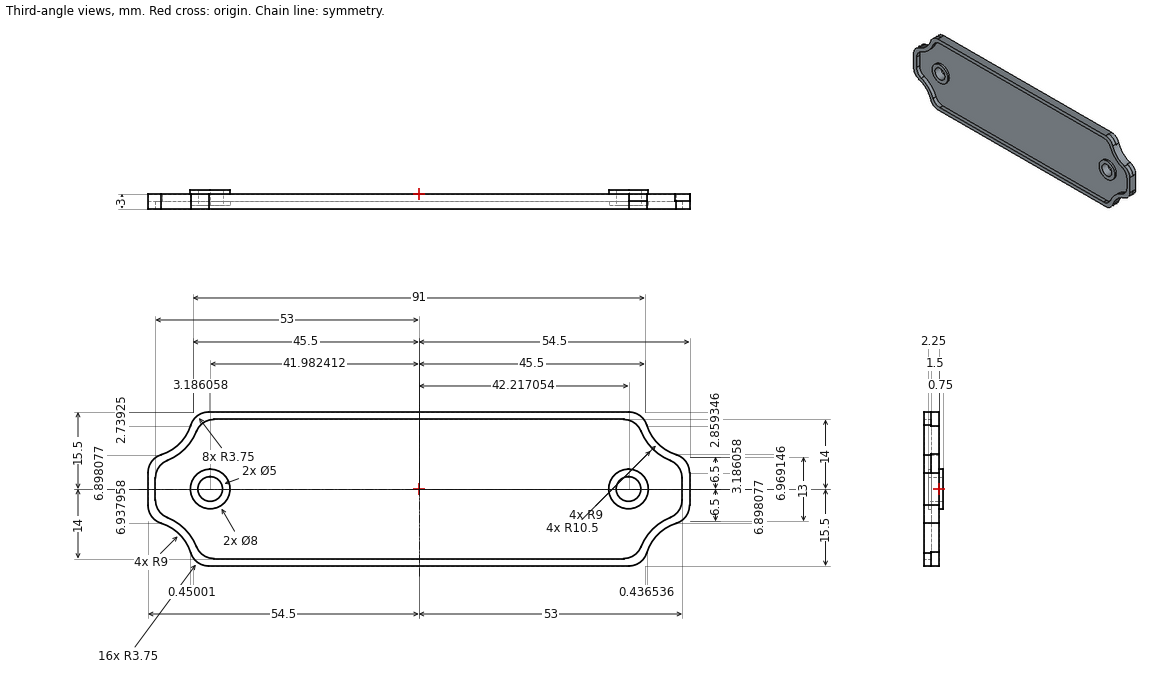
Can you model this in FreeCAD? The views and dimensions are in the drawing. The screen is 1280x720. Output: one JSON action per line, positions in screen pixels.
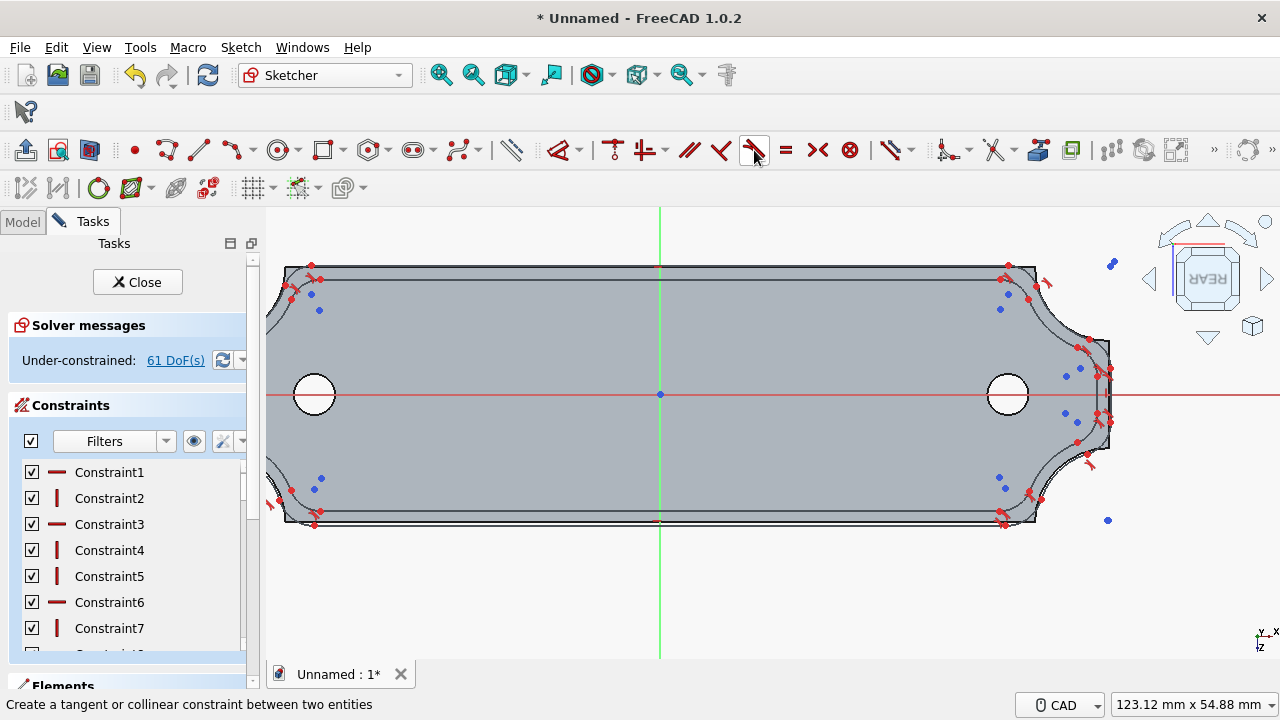
{"action": "left_click", "coordinate": [796, 511]}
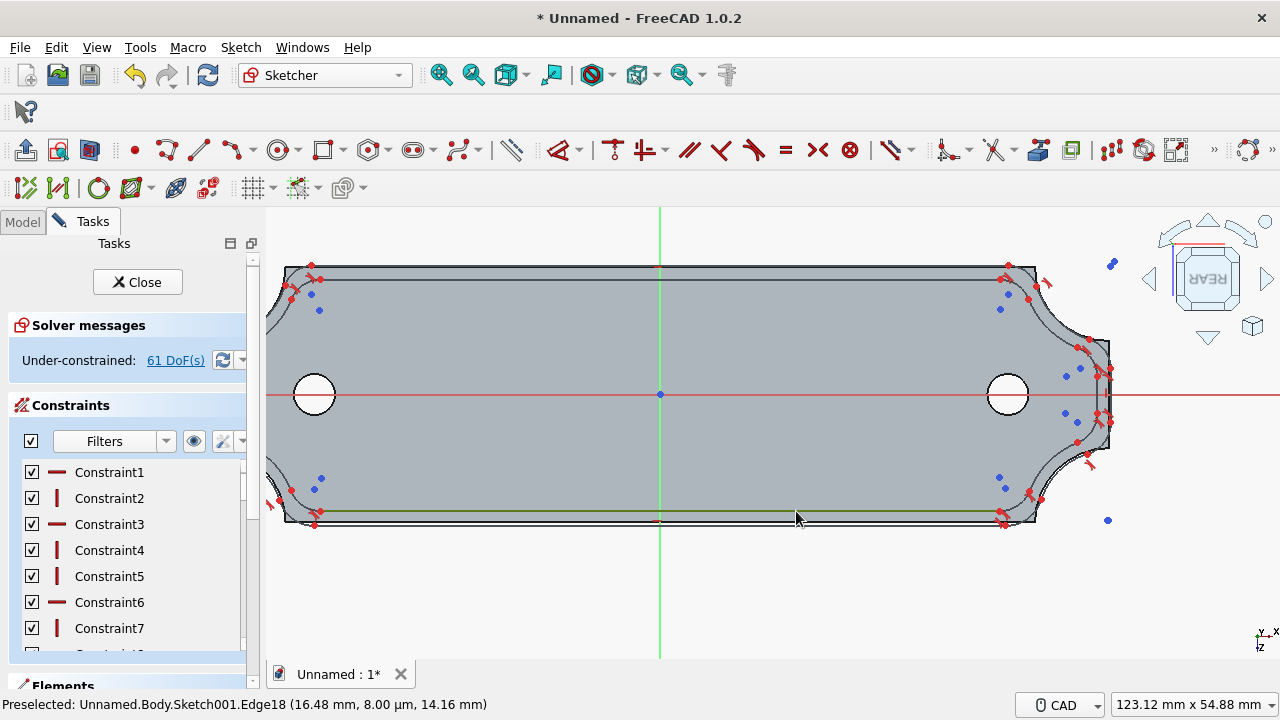
{"action": "scroll", "coordinate": [297, 500], "scroll_direction": "up", "scroll_amount": 2}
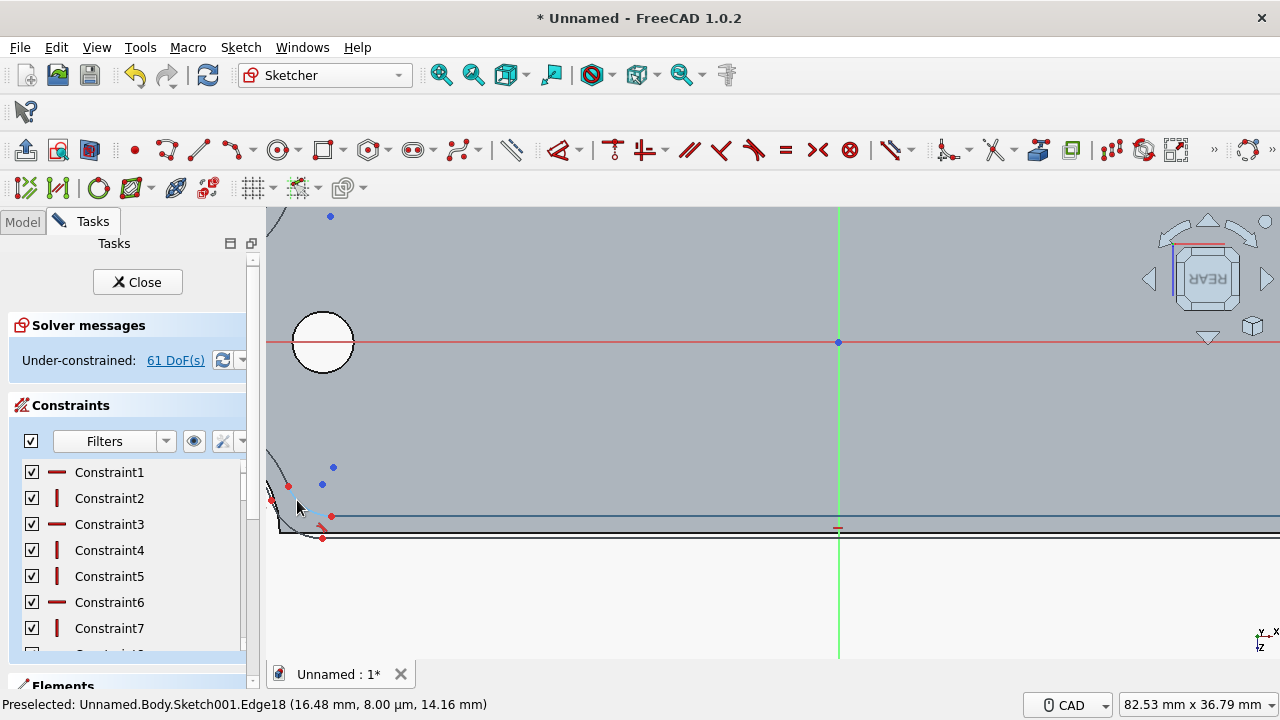
{"action": "left_click", "coordinate": [297, 500]}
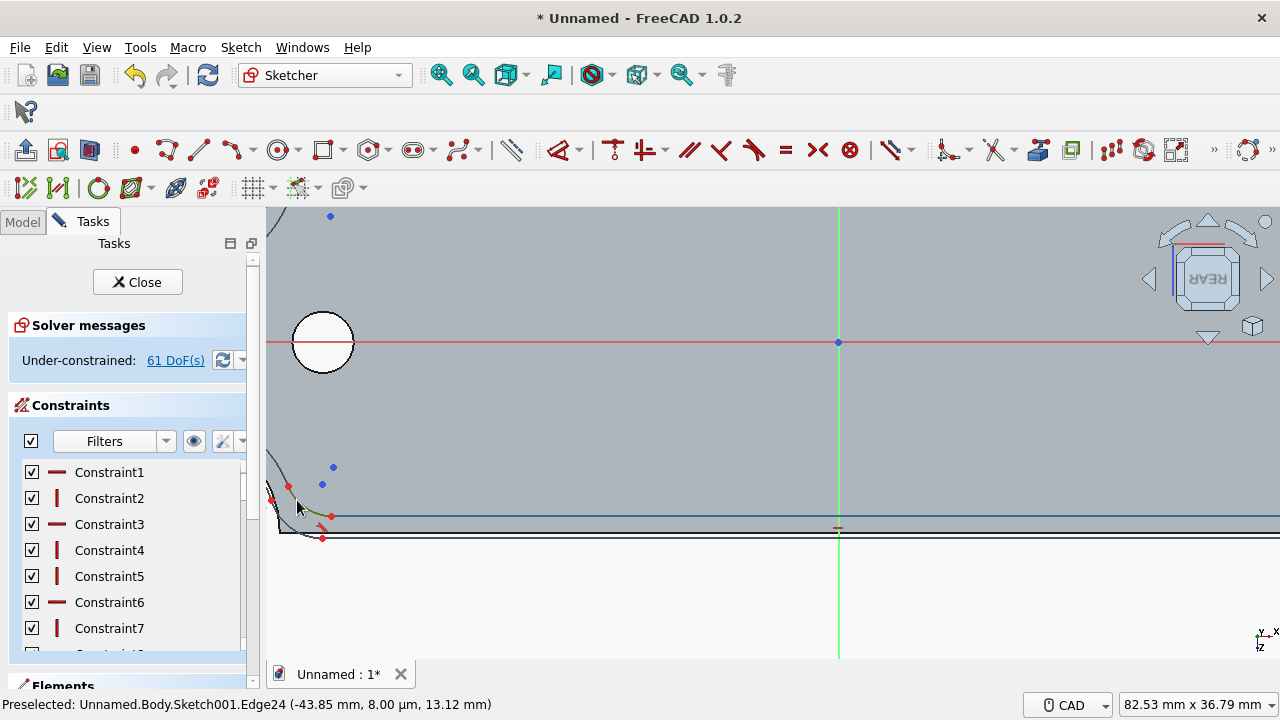
{"action": "left_click", "coordinate": [754, 150]}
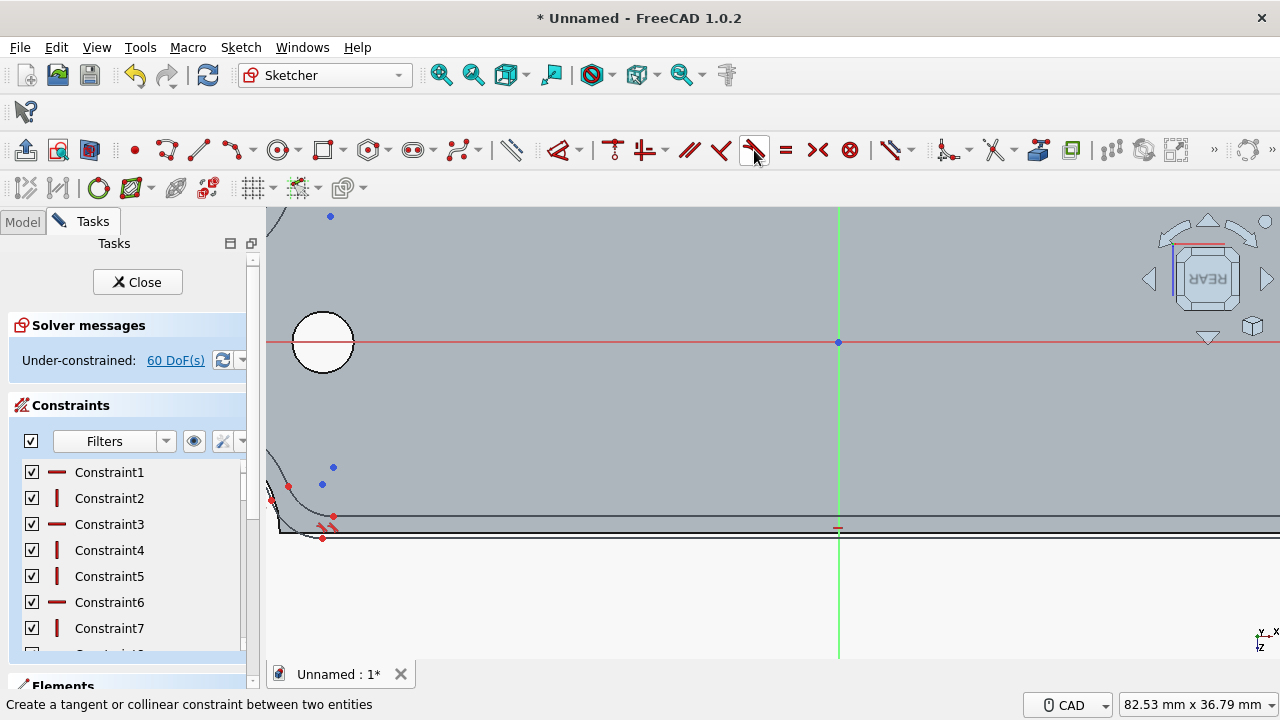
{"action": "scroll", "coordinate": [595, 507], "scroll_direction": "down", "scroll_amount": 4}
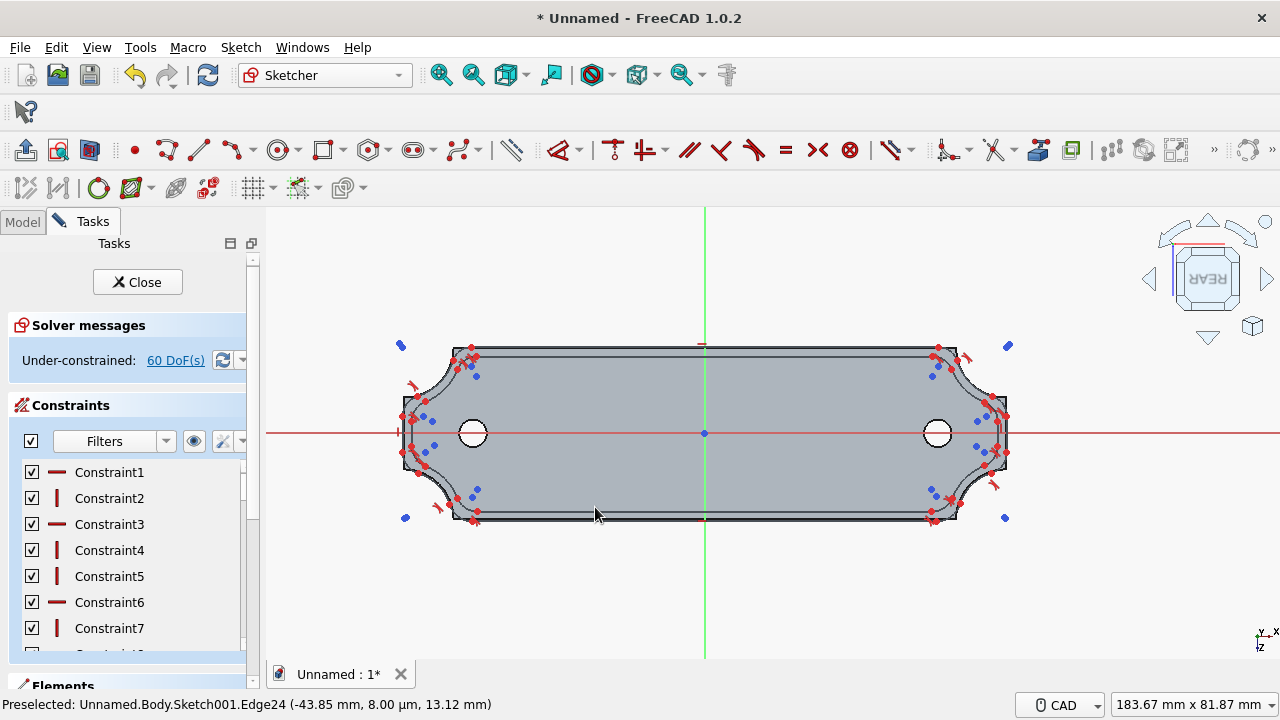
{"action": "scroll", "coordinate": [412, 439], "scroll_direction": "up", "scroll_amount": 5}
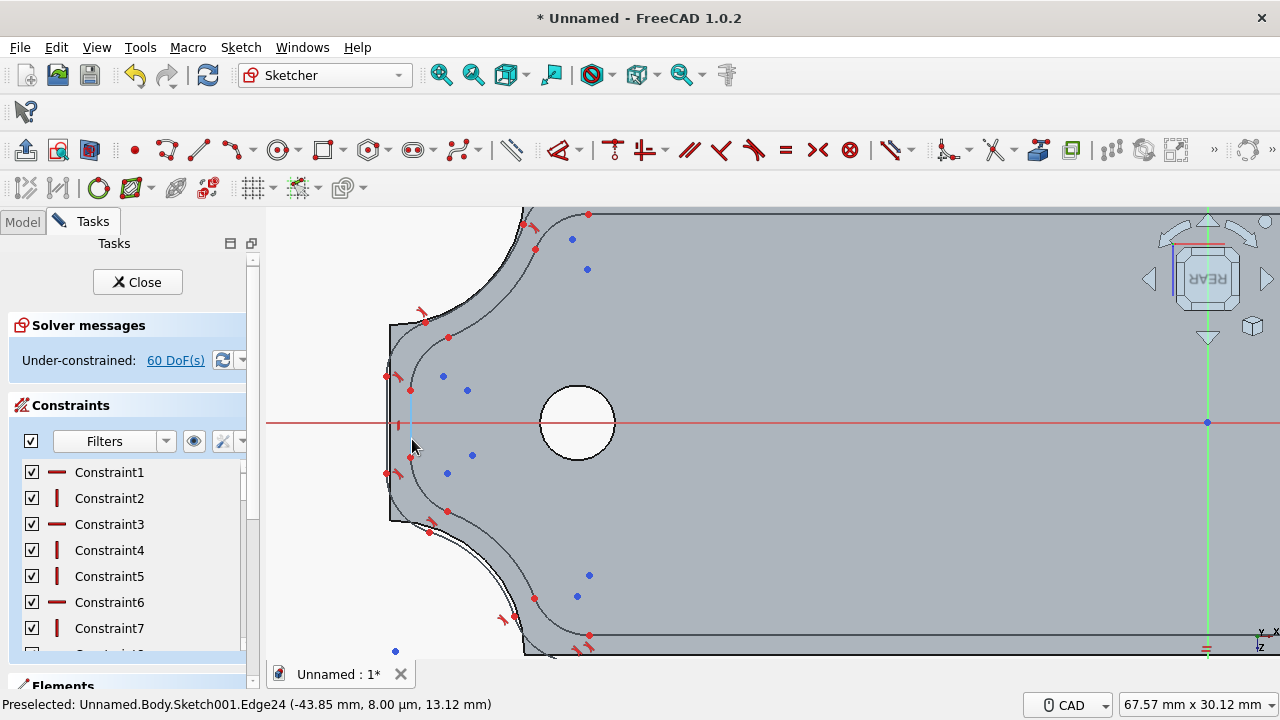
{"action": "left_click", "coordinate": [411, 437]}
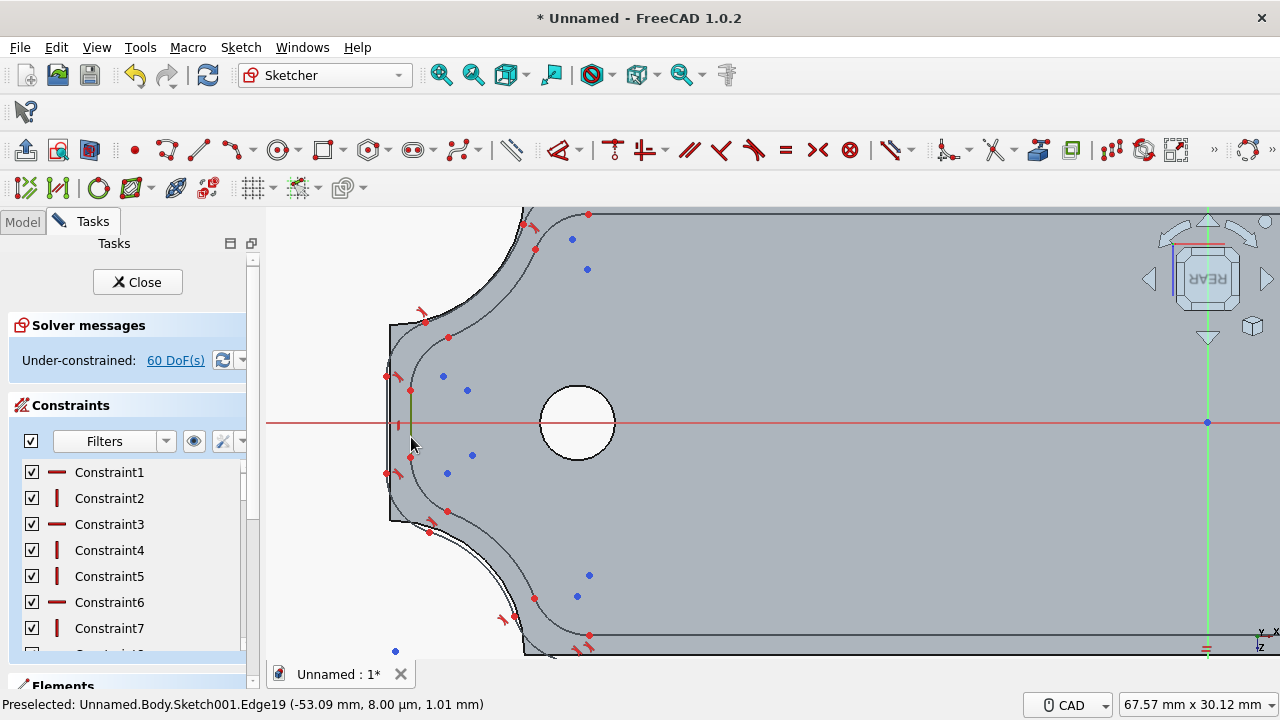
{"action": "left_click", "coordinate": [415, 478]}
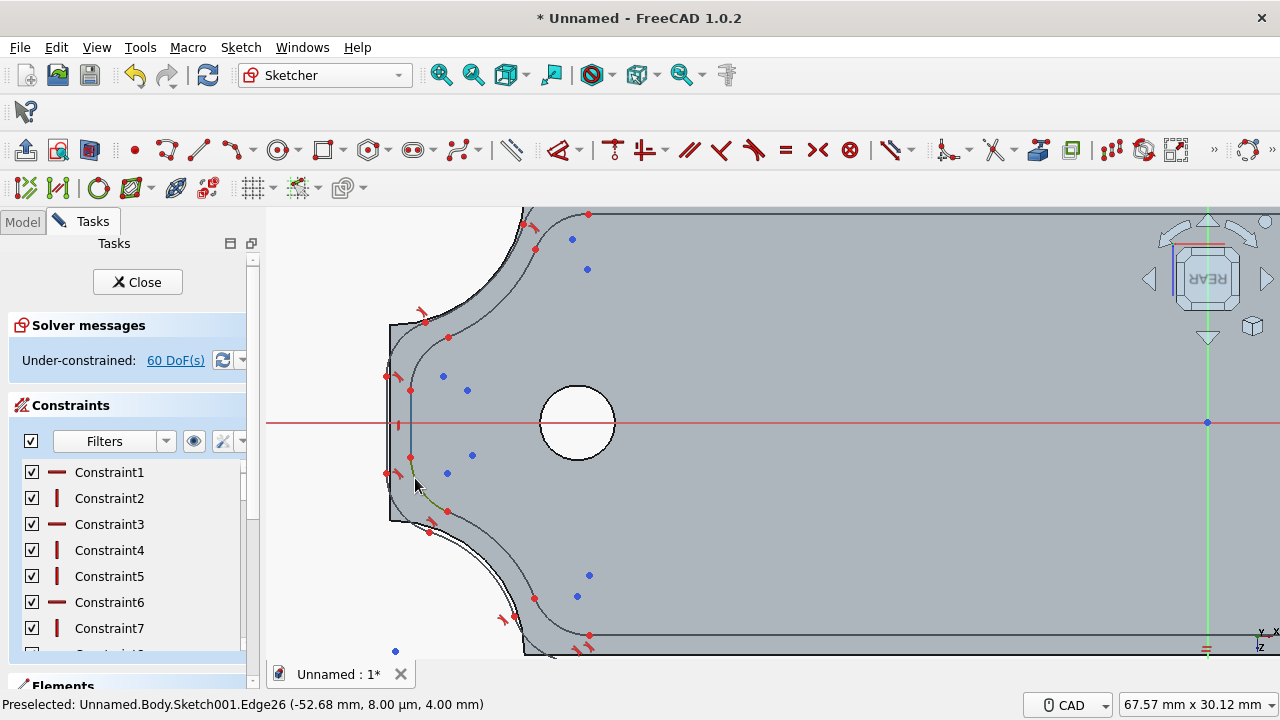
{"action": "left_click", "coordinate": [754, 150]}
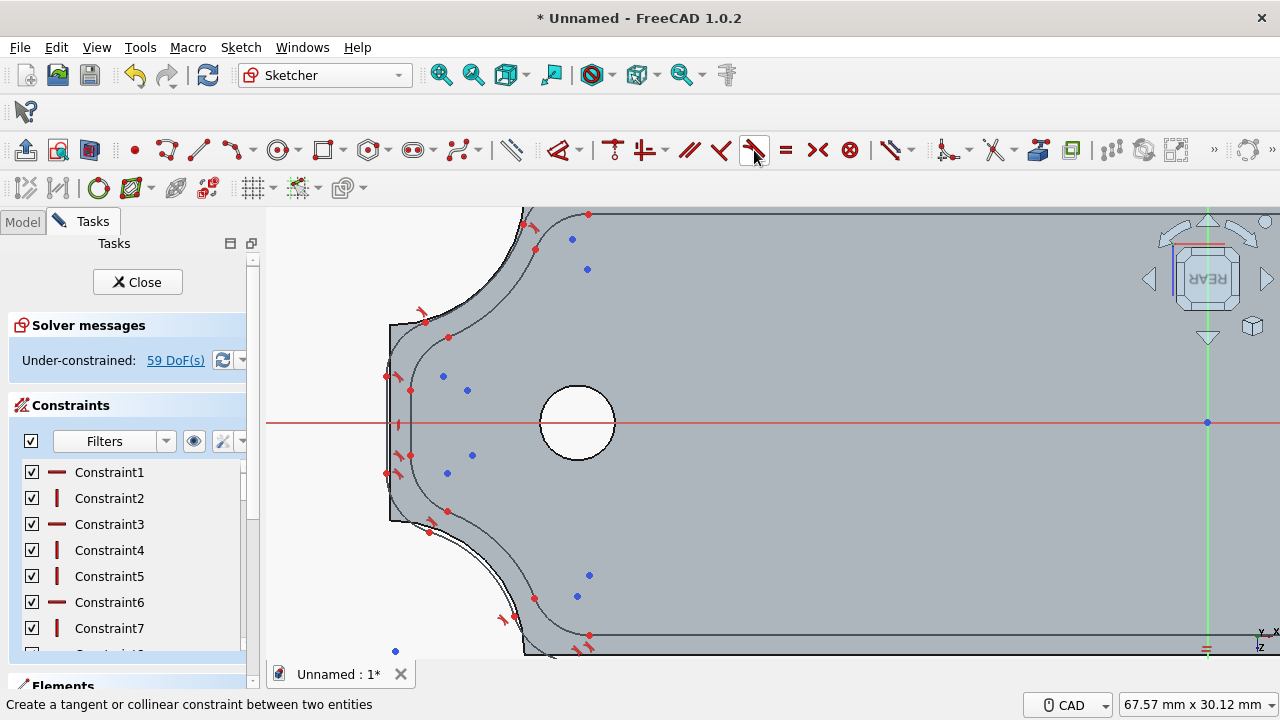
{"action": "left_click", "coordinate": [411, 436]}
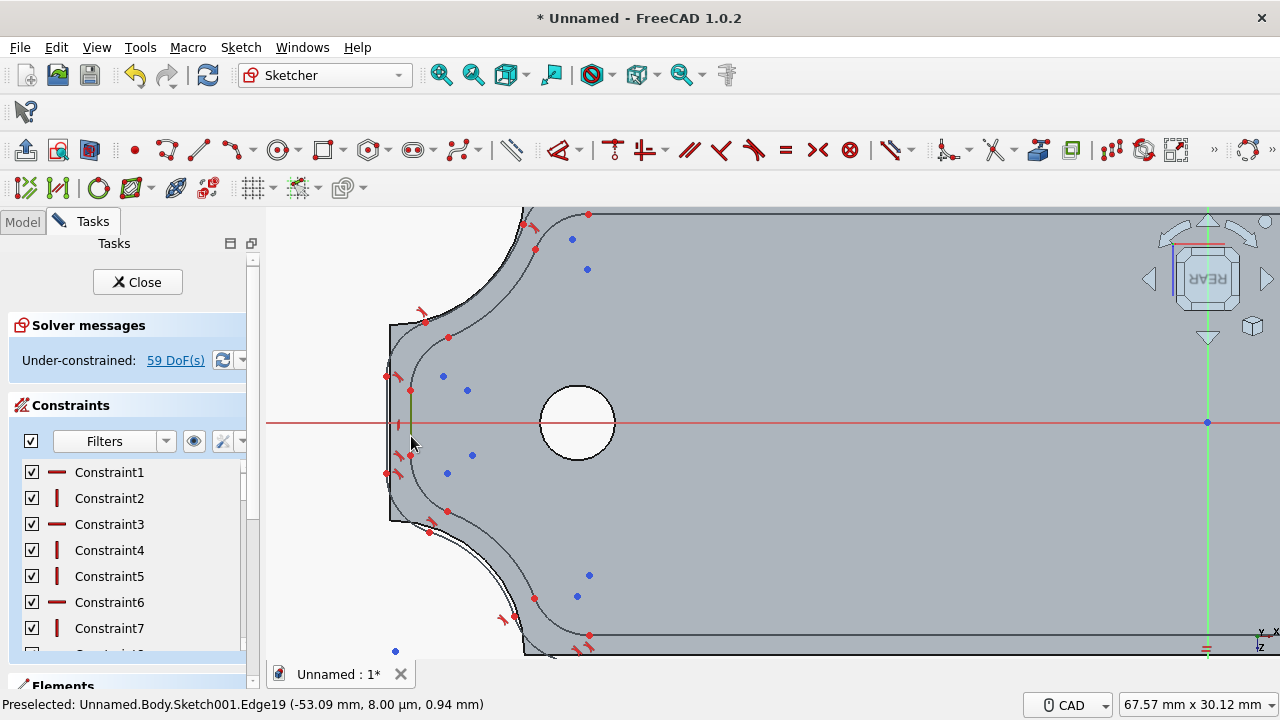
{"action": "left_click", "coordinate": [430, 348]}